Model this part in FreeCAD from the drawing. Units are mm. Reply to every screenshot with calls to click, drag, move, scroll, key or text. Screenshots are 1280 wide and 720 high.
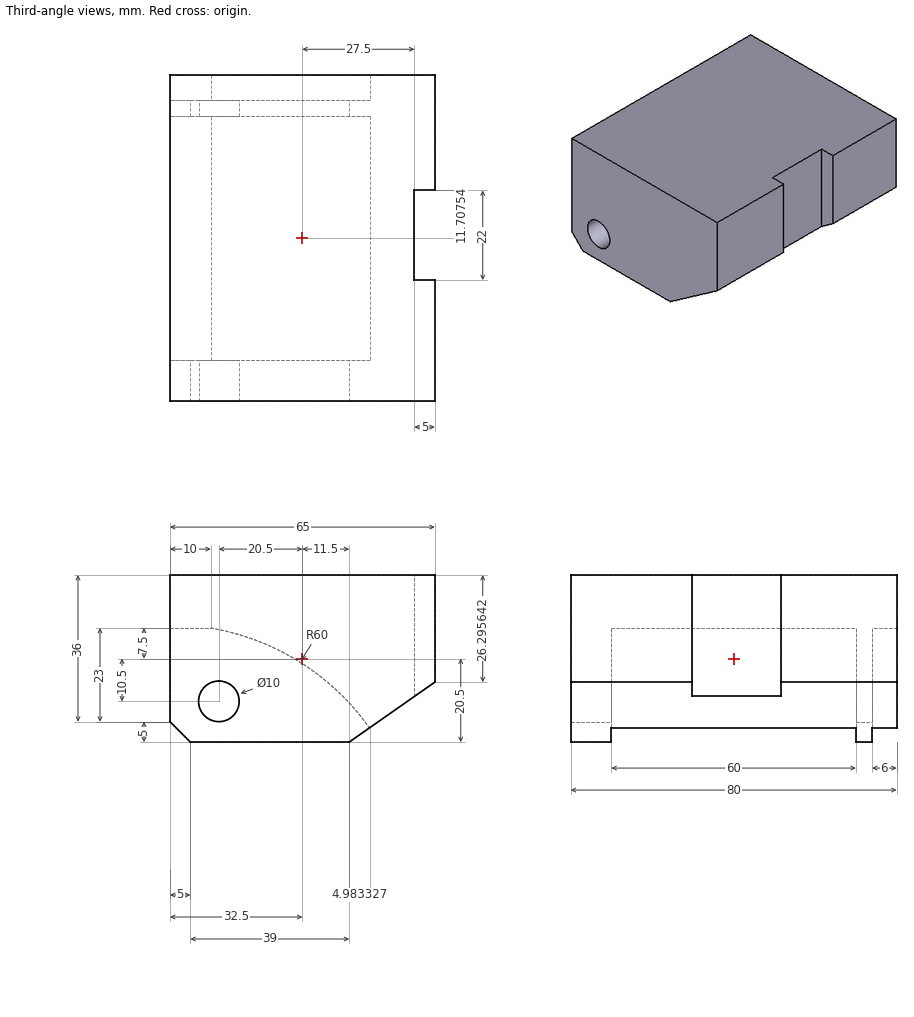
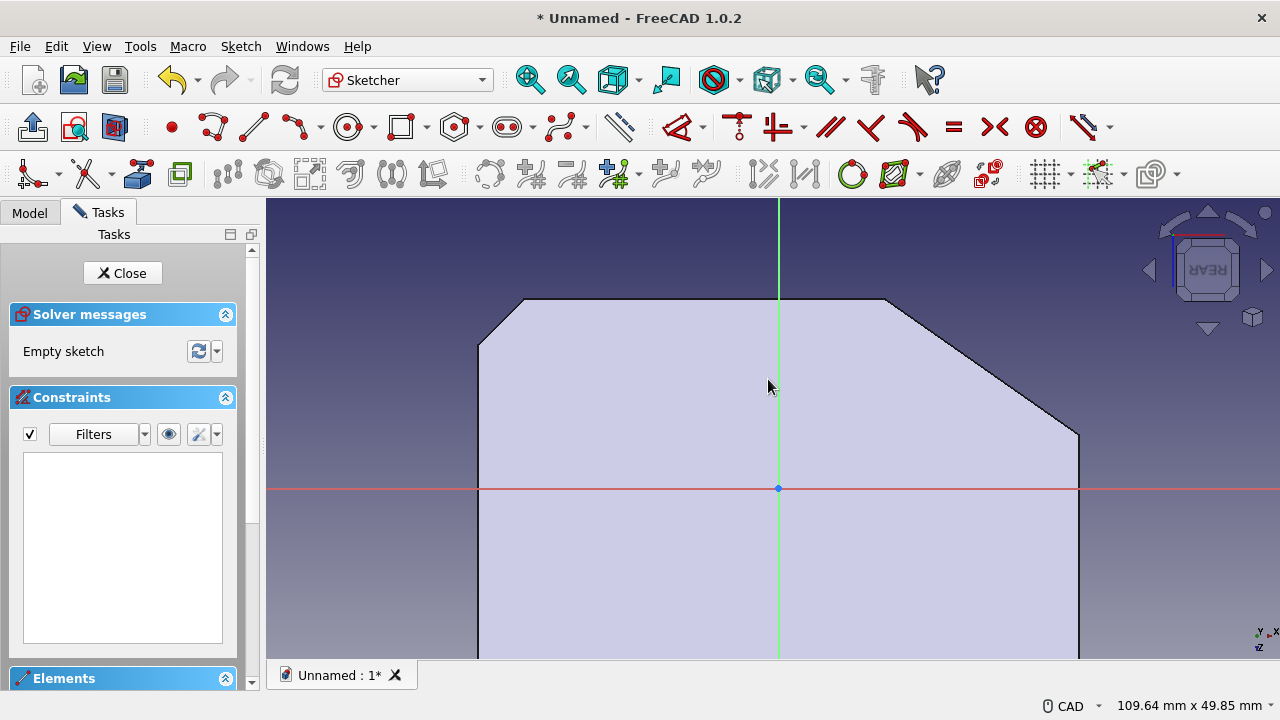
click(213, 128)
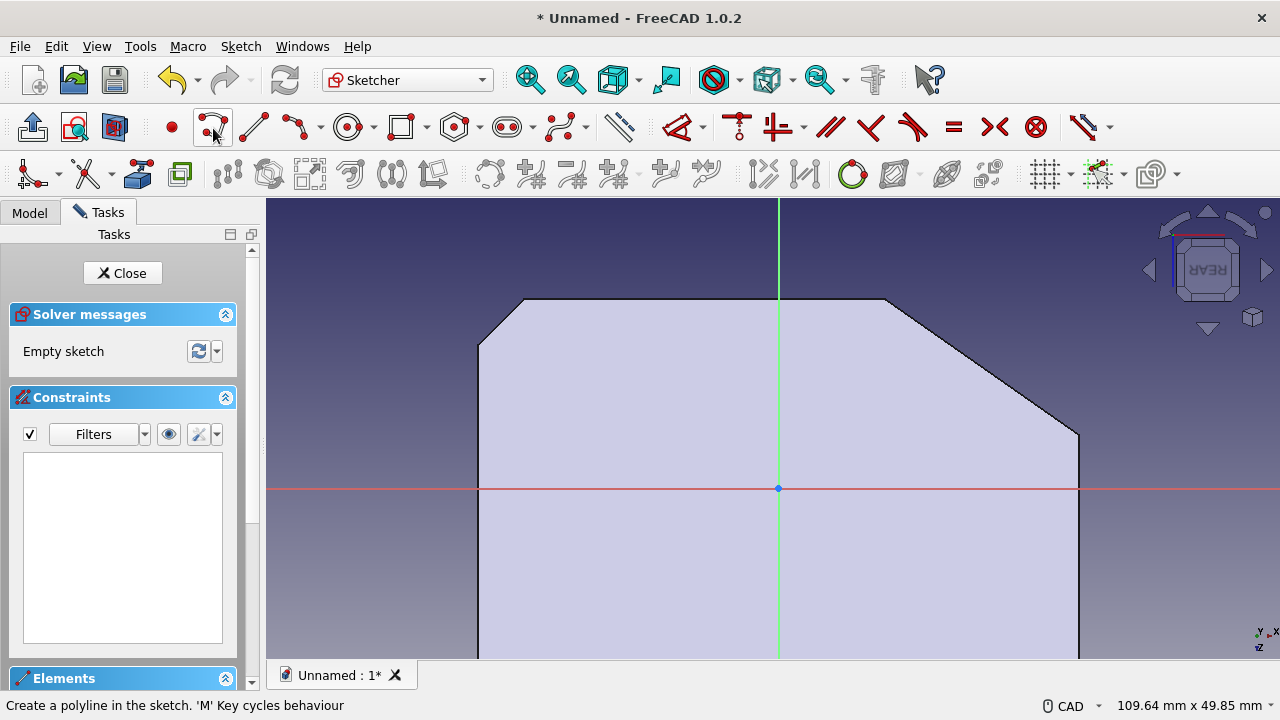
click(931, 331)
click(885, 299)
click(524, 299)
click(478, 345)
click(478, 558)
click(570, 558)
right_click(570, 558)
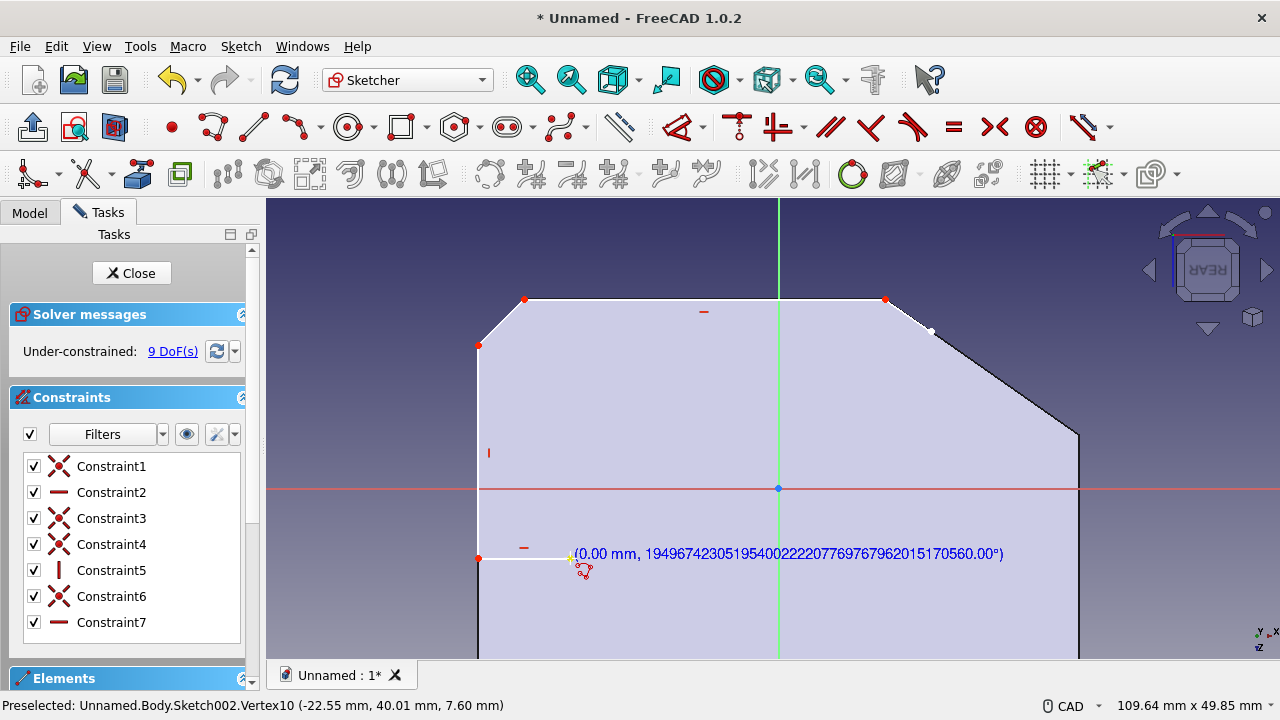
click(294, 128)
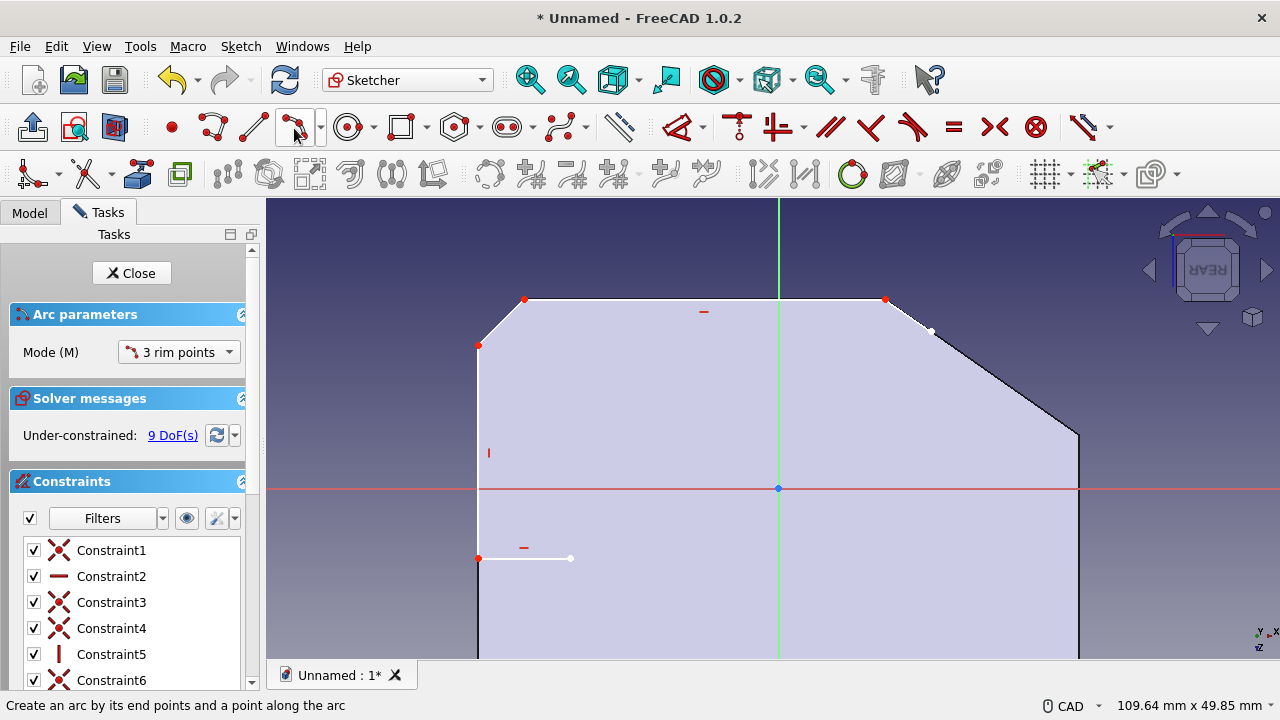
click(570, 559)
click(931, 332)
click(809, 456)
key(Escape)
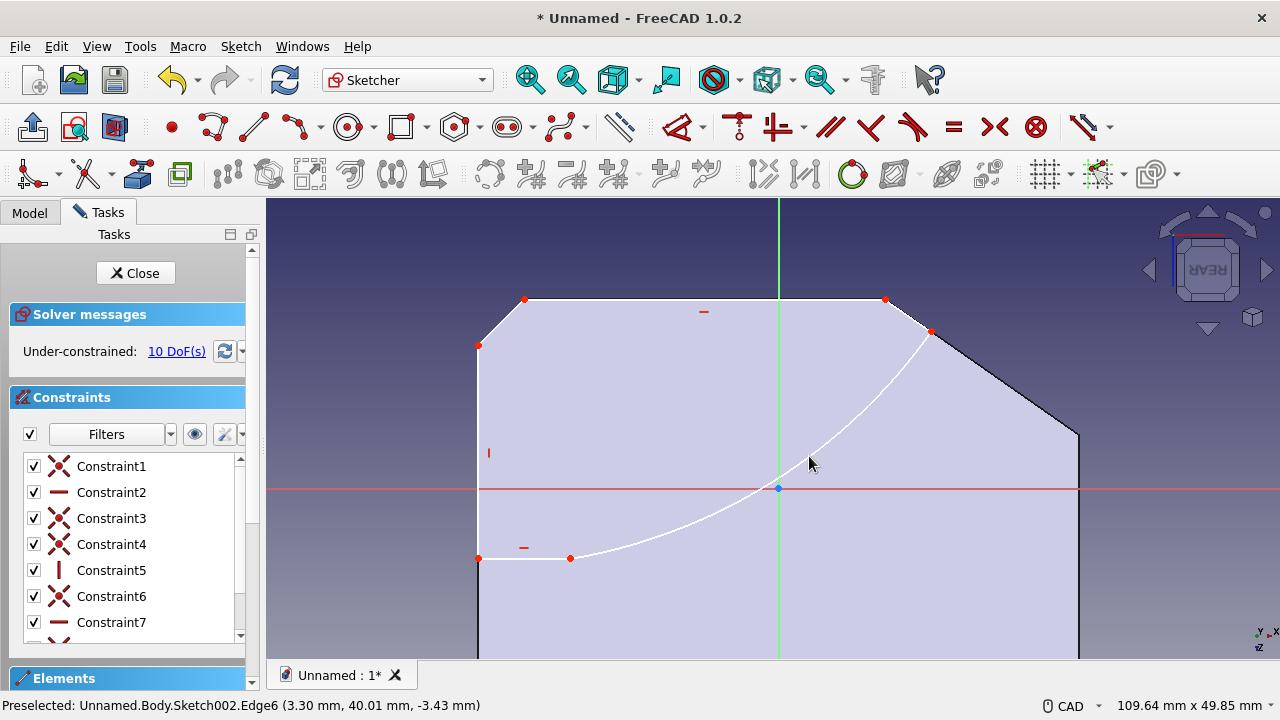
key(d)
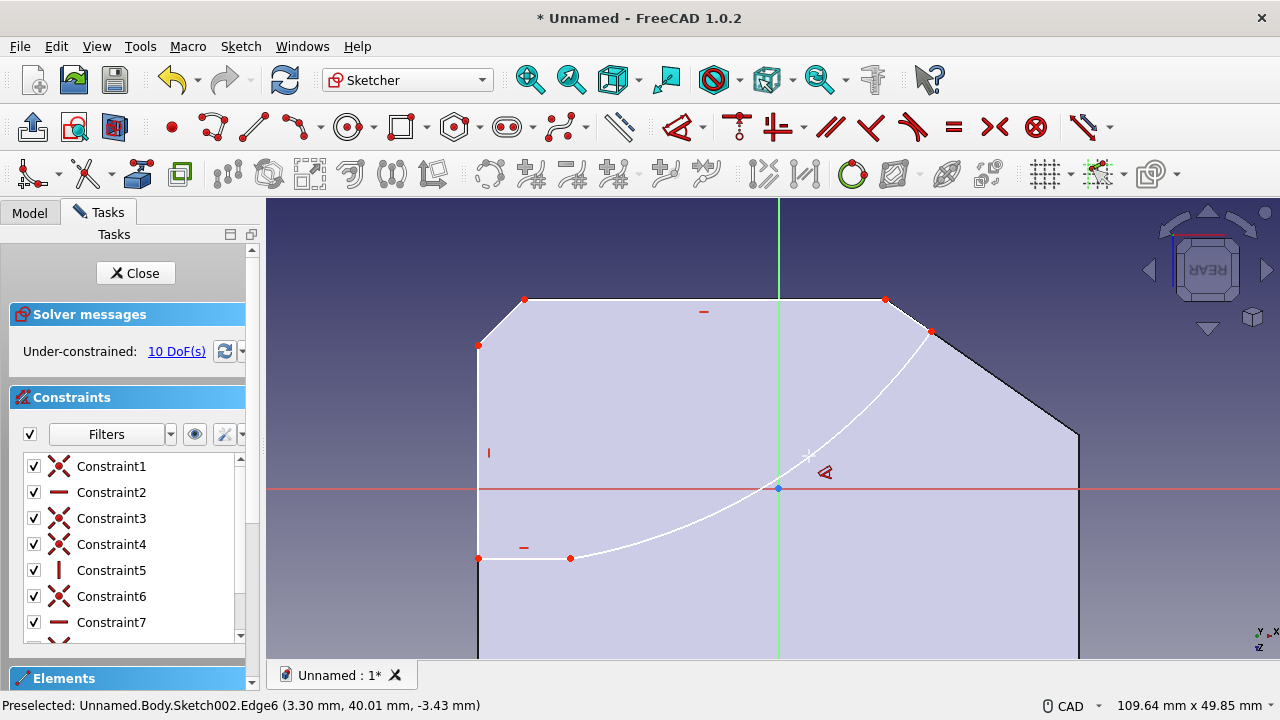
click(696, 522)
click(709, 551)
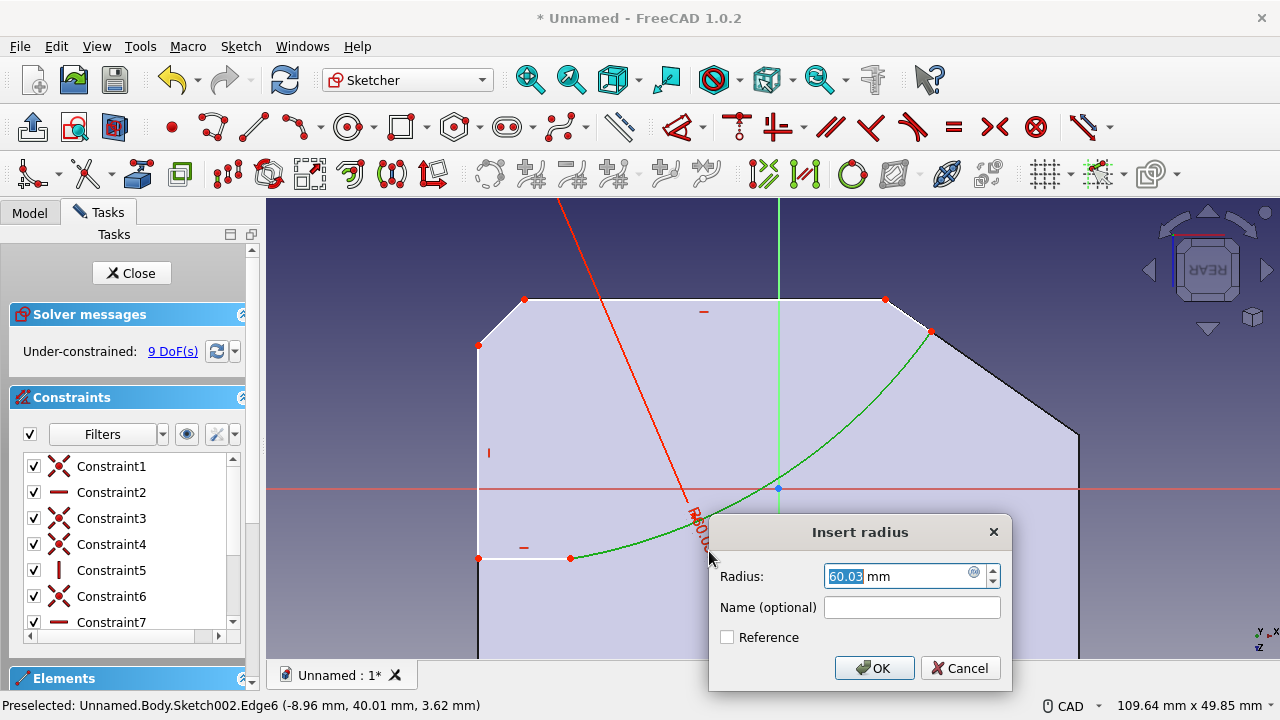
text(60)
key(Return)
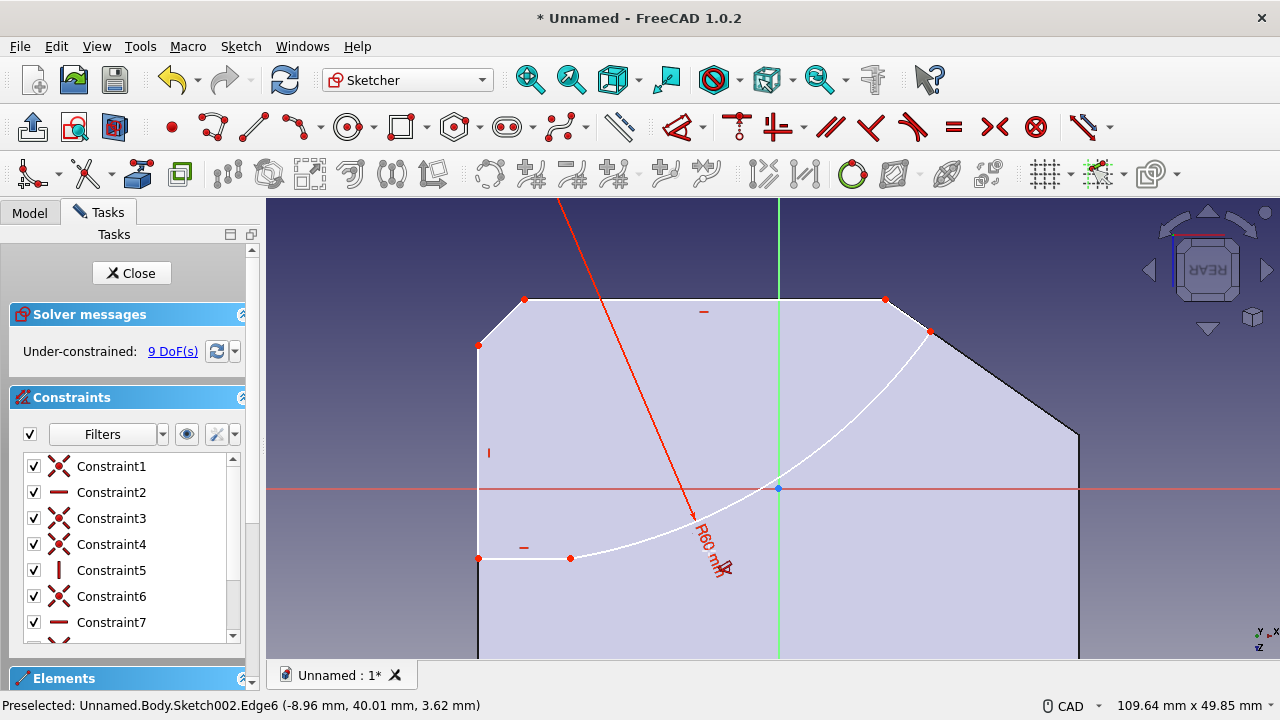
click(777, 300)
click(705, 266)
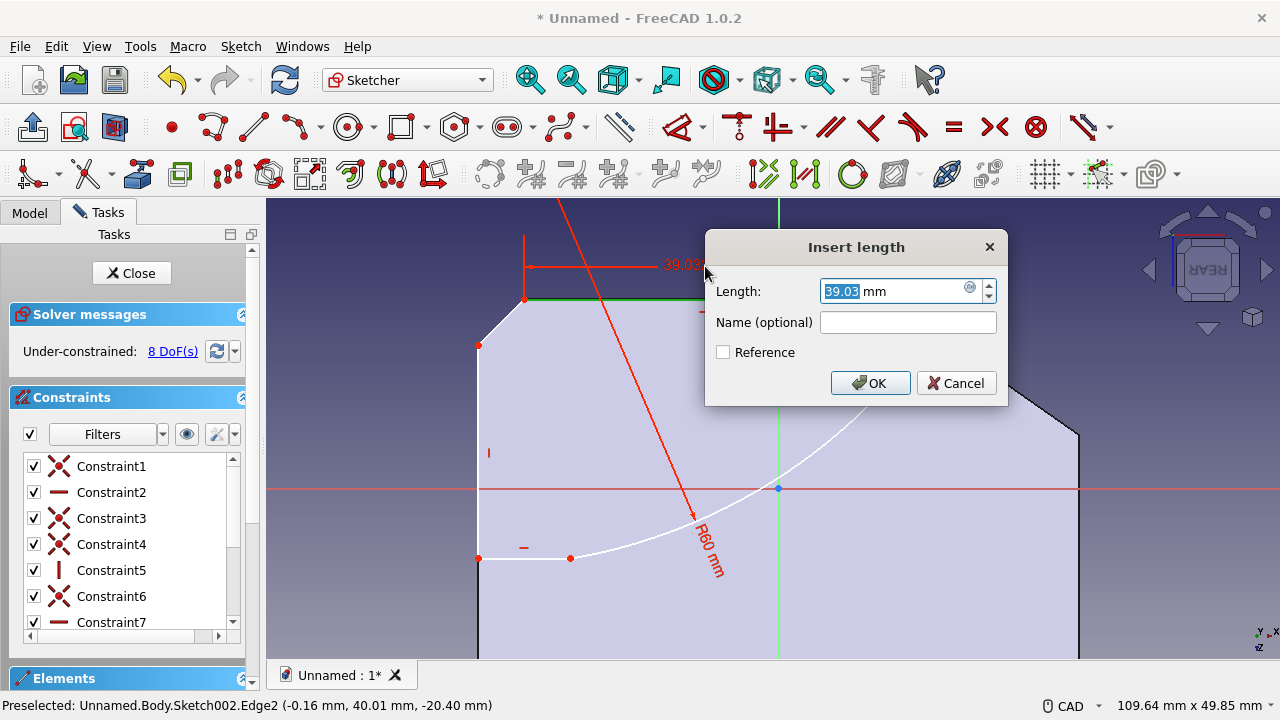
text(39)
key(Return)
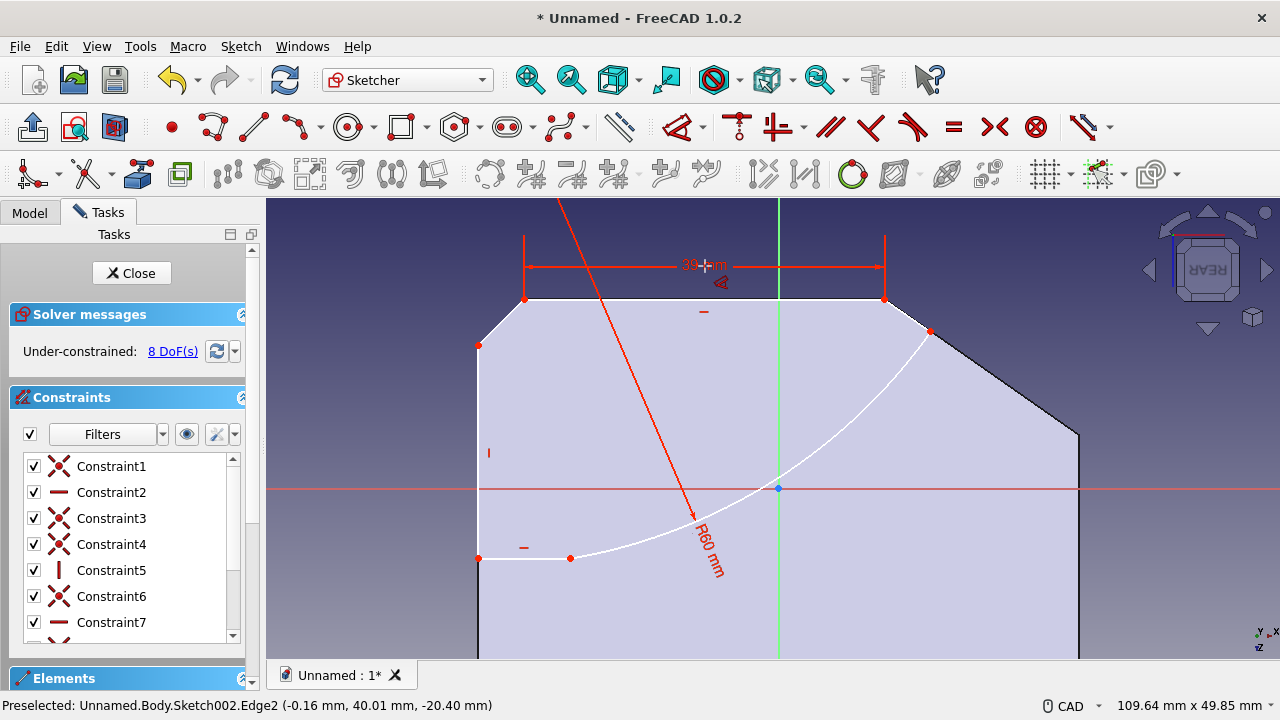
click(478, 410)
click(444, 452)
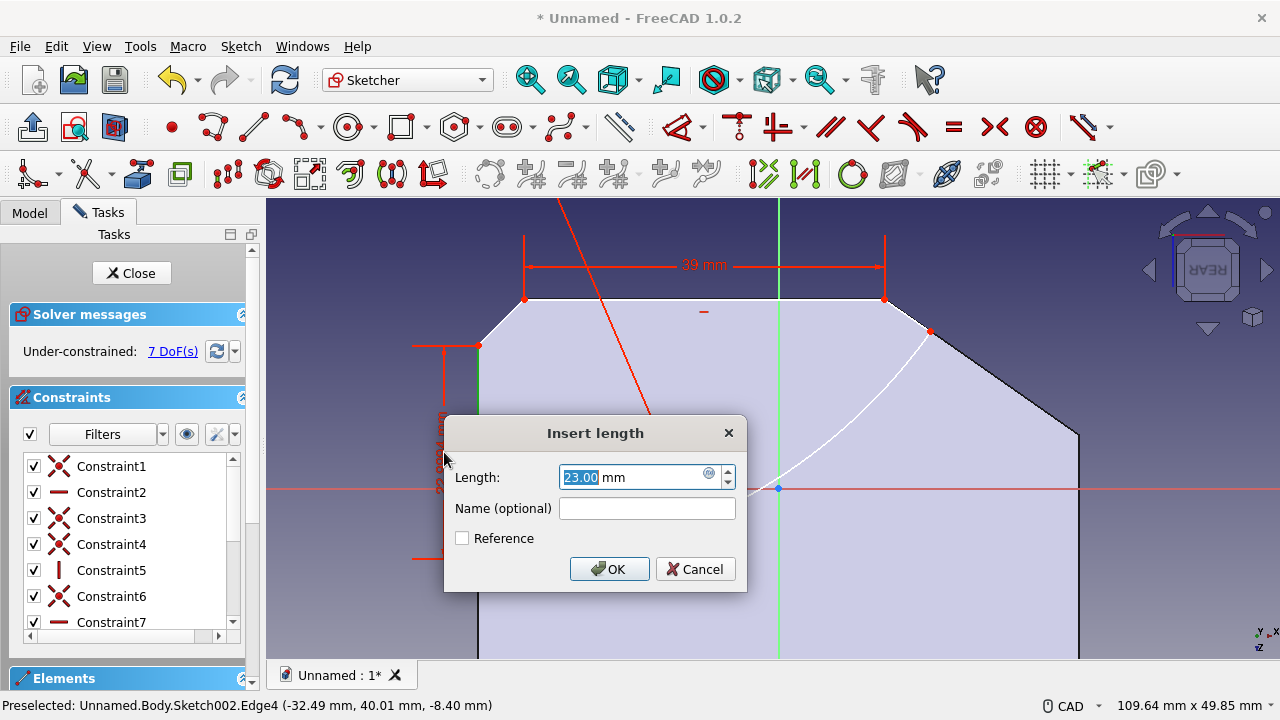
text(23)
key(Return)